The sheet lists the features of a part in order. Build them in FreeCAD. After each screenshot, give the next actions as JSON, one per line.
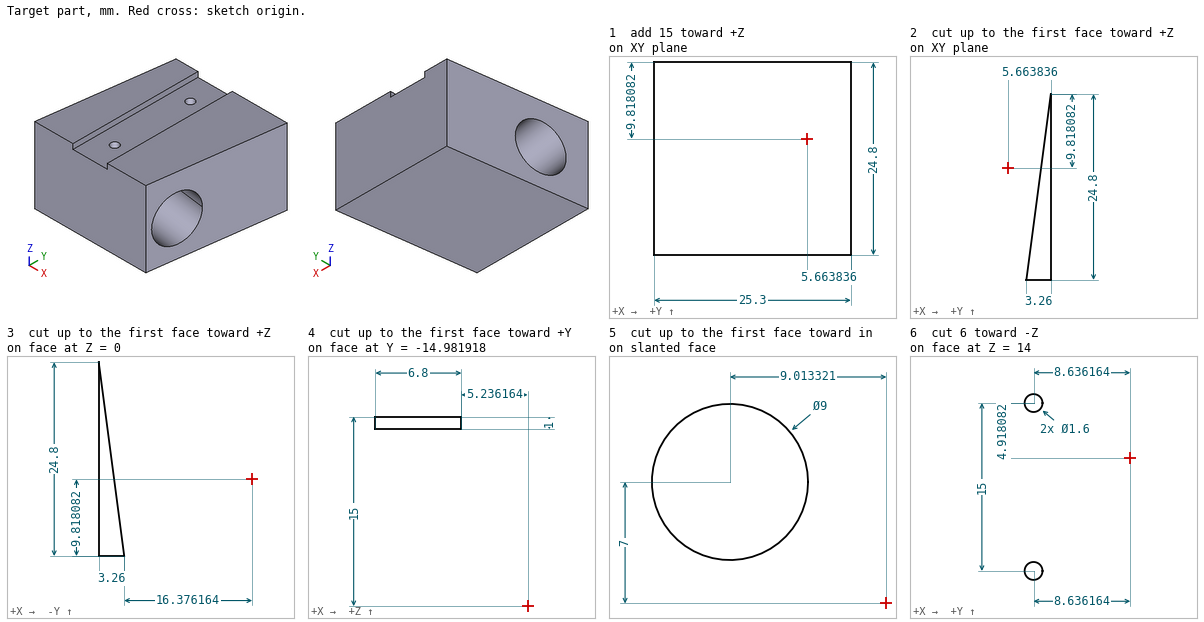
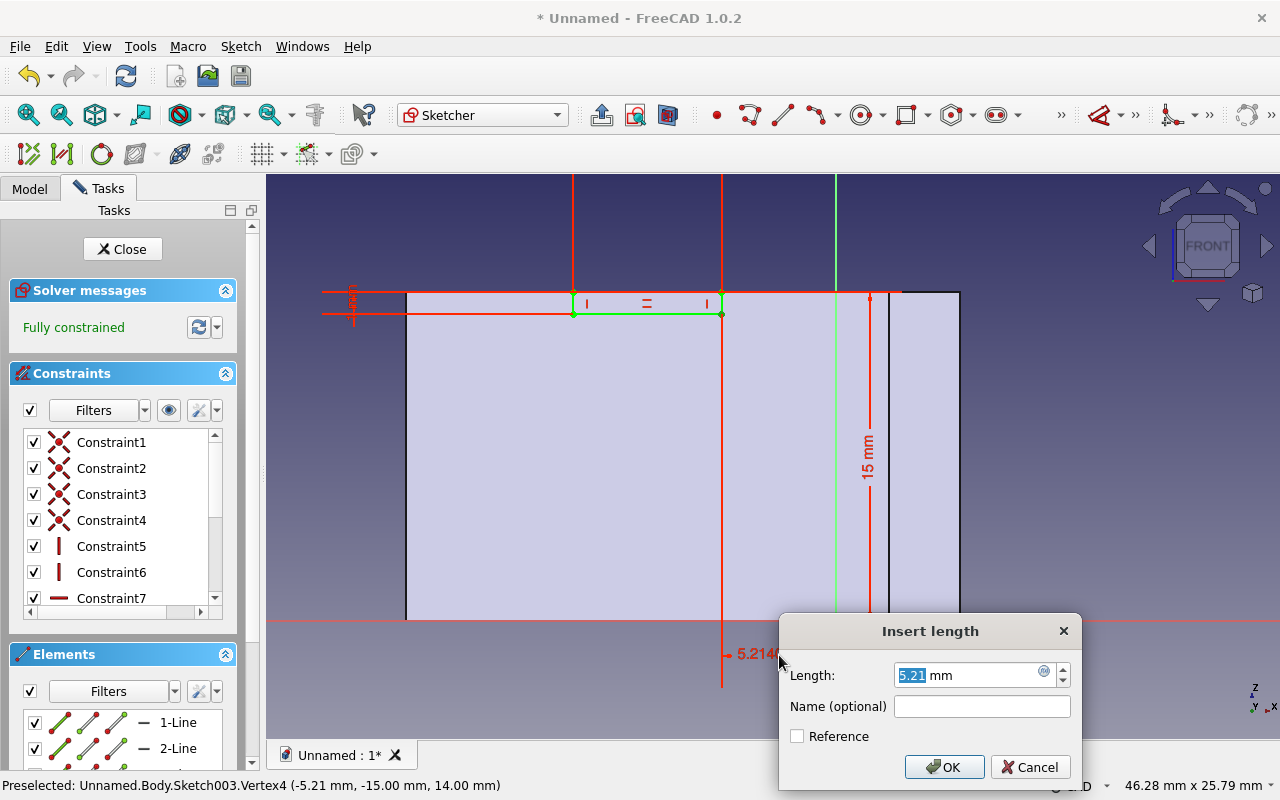
{"action": "type", "text": "5.236164"}
{"action": "key", "text": "Return"}
{"action": "key", "text": "Escape"}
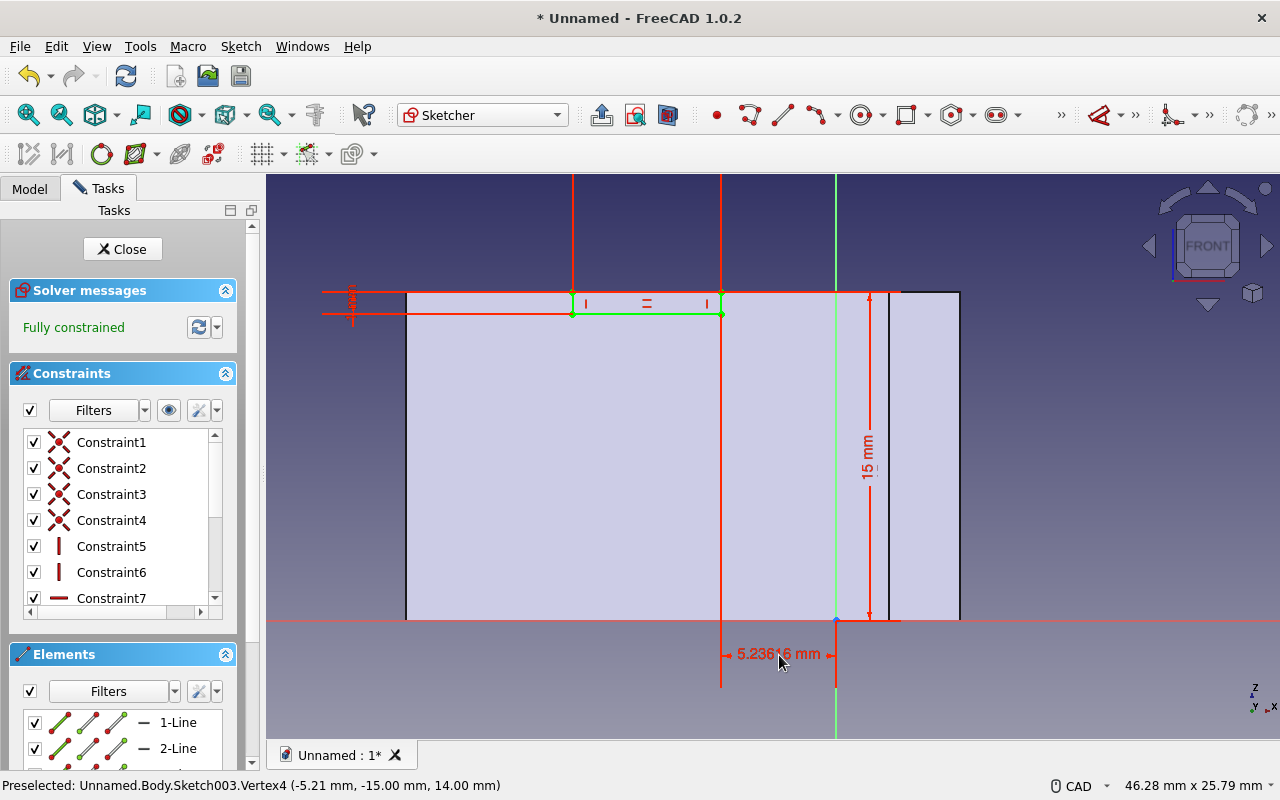
{"action": "left_click", "coordinate": [123, 249]}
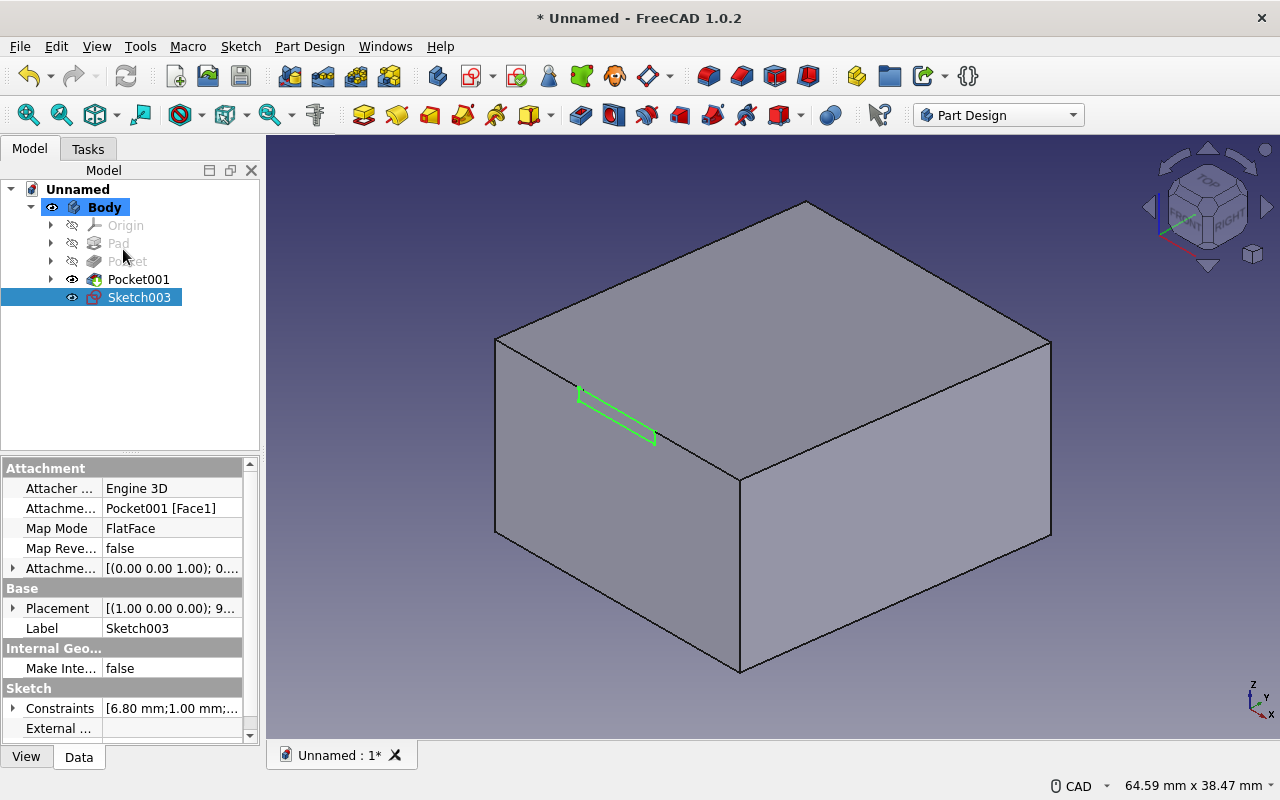
{"action": "left_click", "coordinate": [581, 116]}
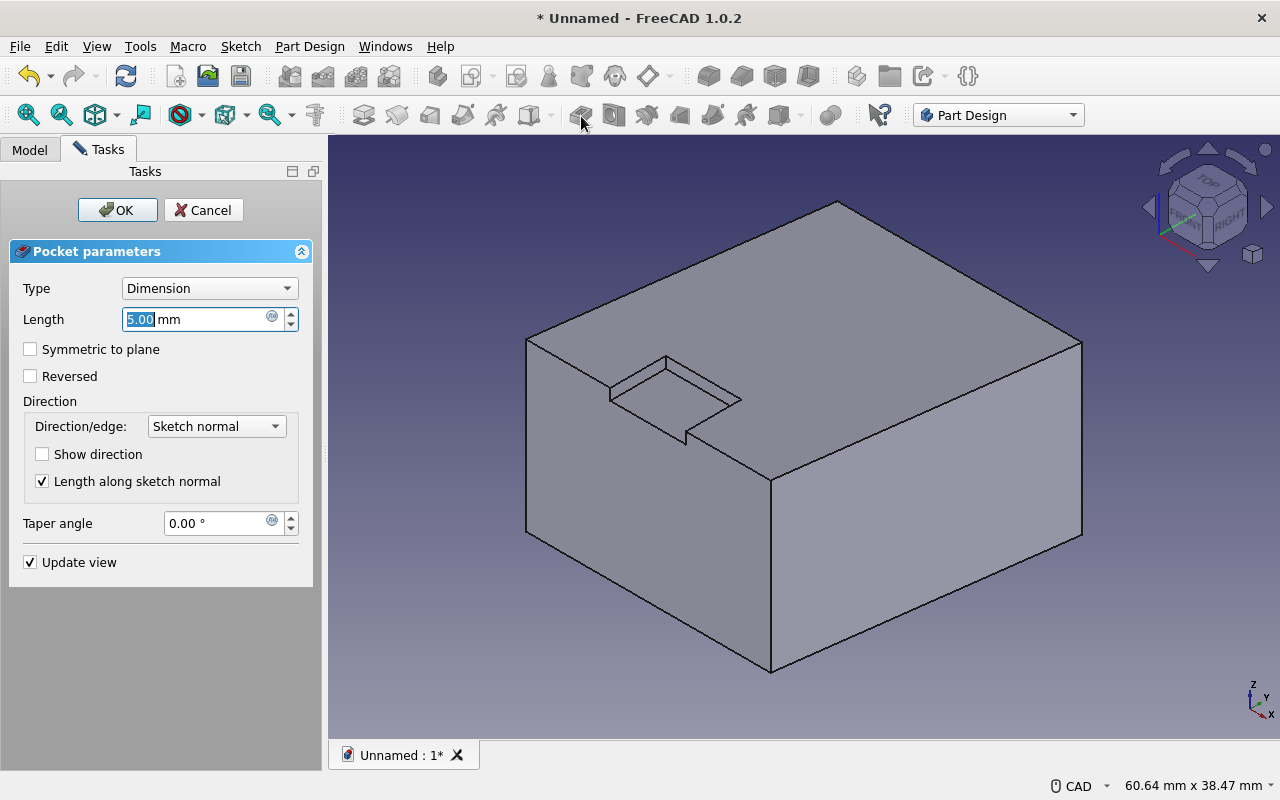
{"action": "left_click", "coordinate": [210, 288]}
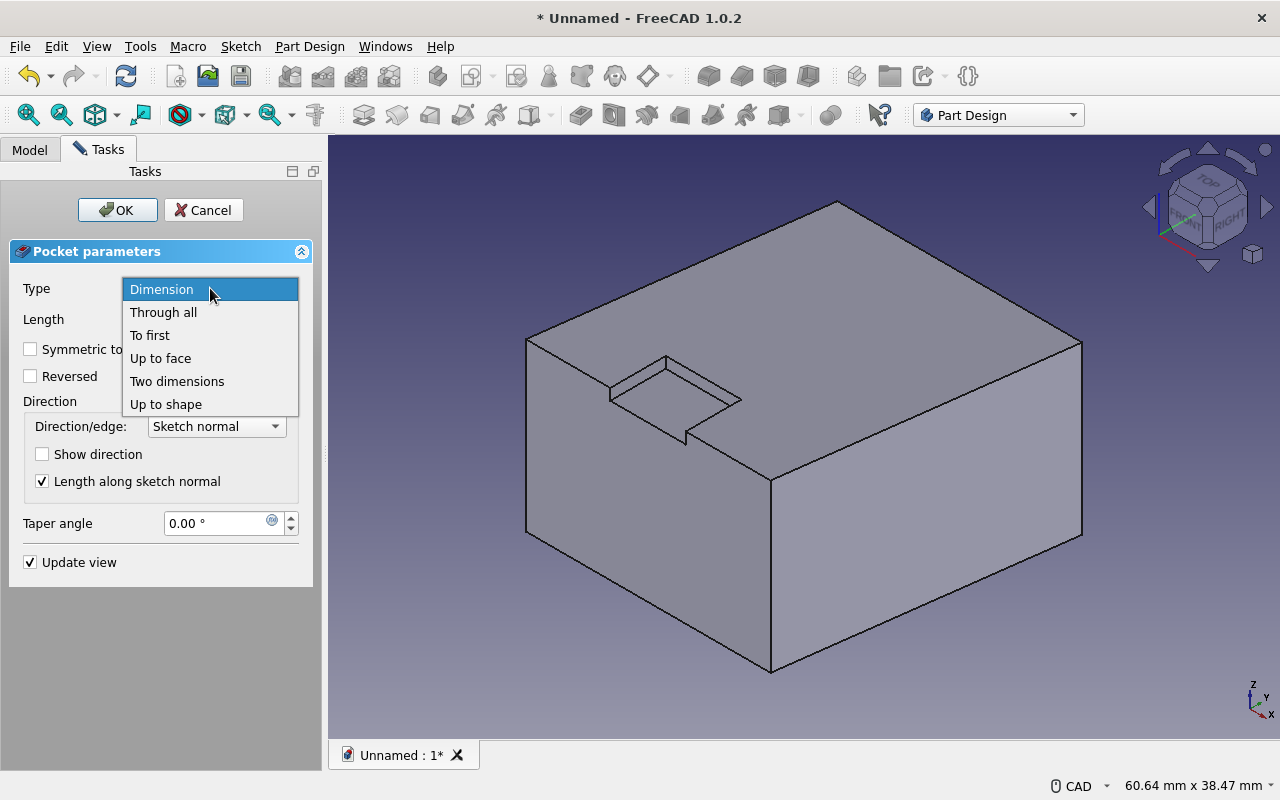
{"action": "left_click", "coordinate": [208, 336]}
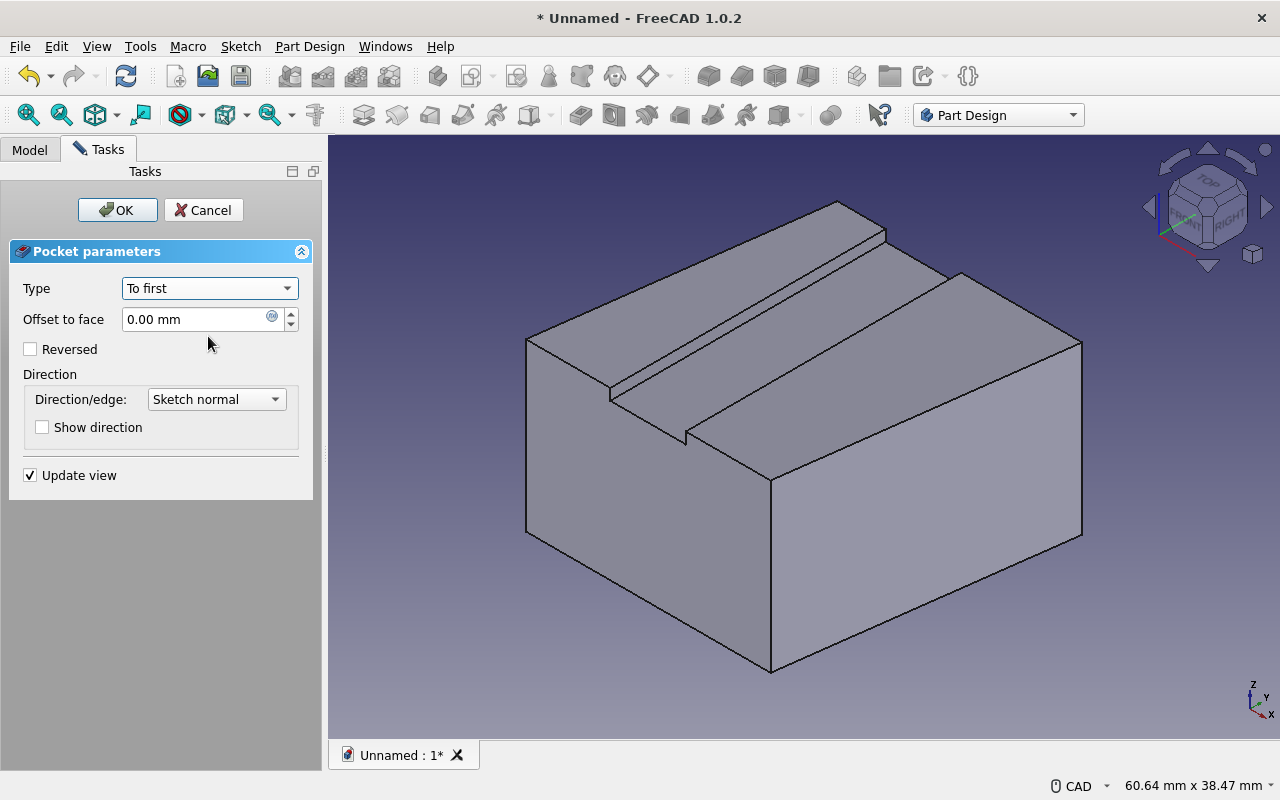
{"action": "left_click", "coordinate": [118, 210]}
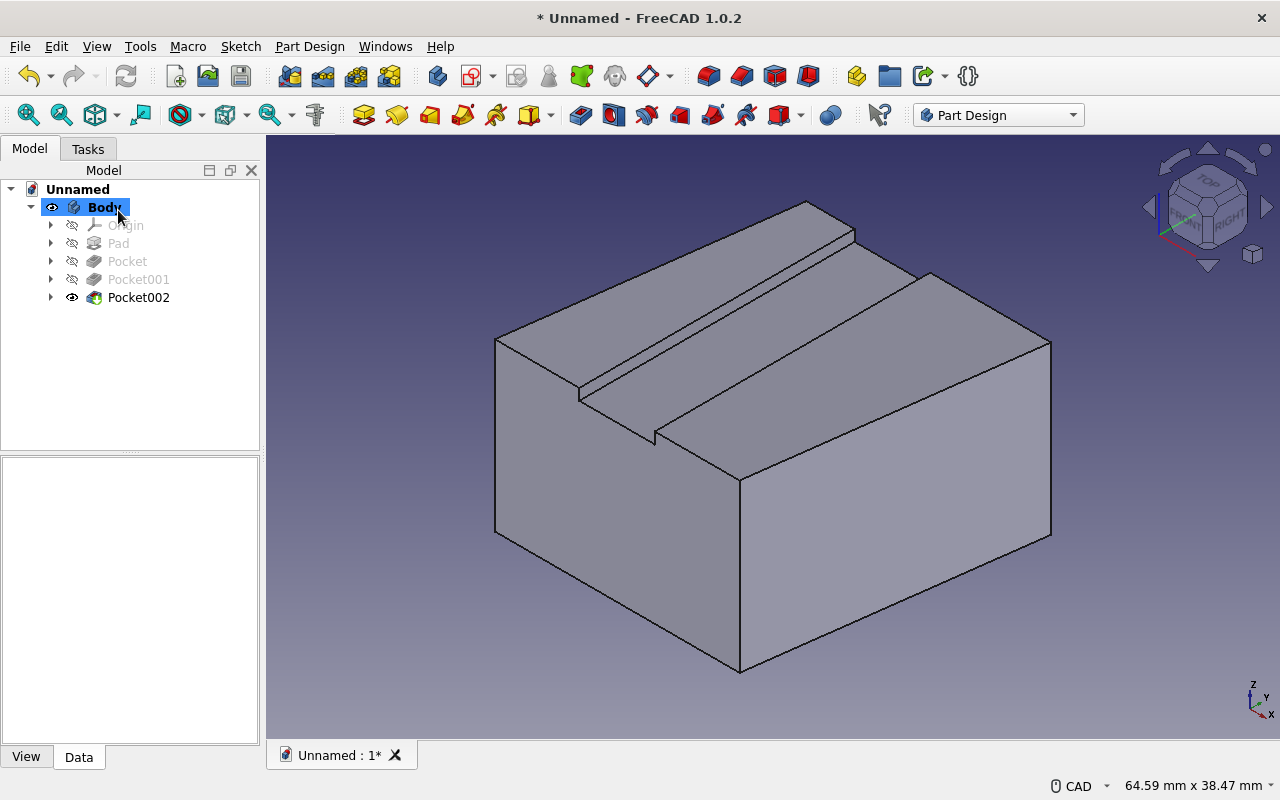
{"action": "left_click", "coordinate": [940, 487]}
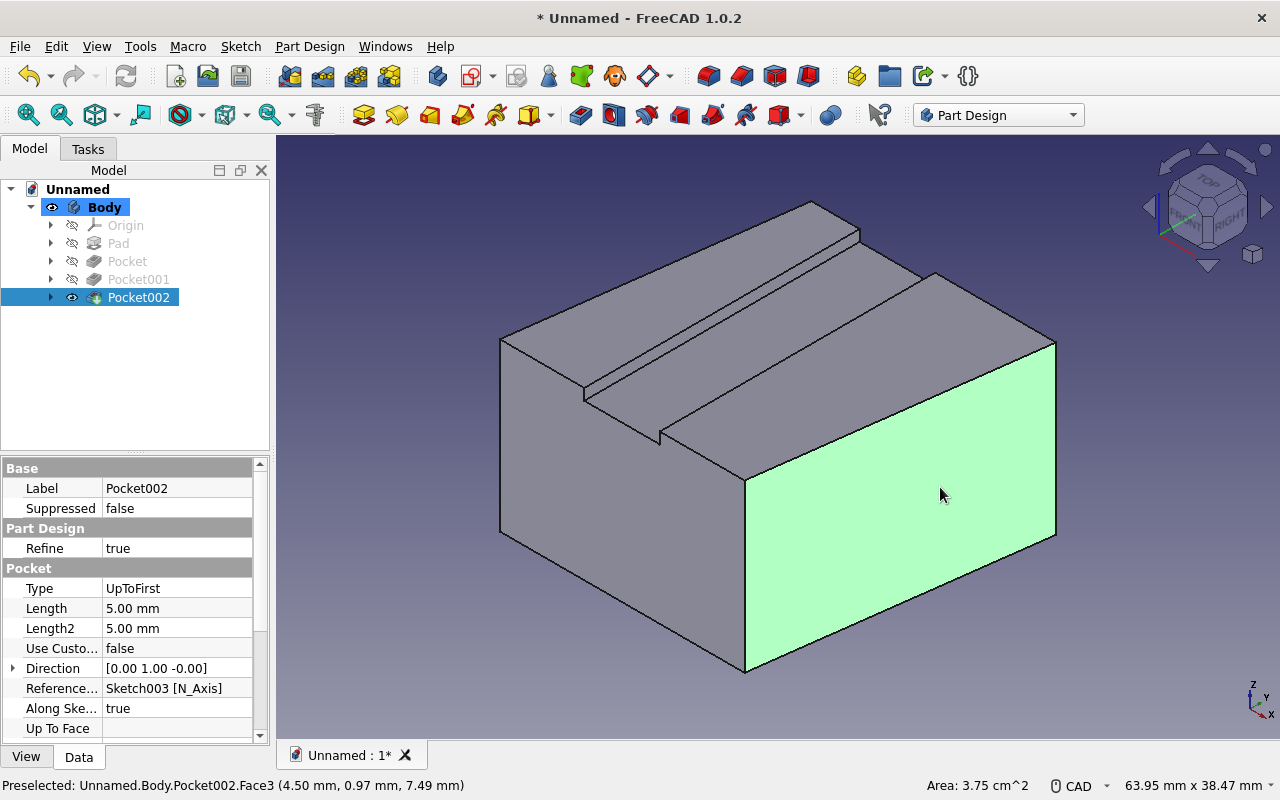
{"action": "left_click", "coordinate": [470, 76]}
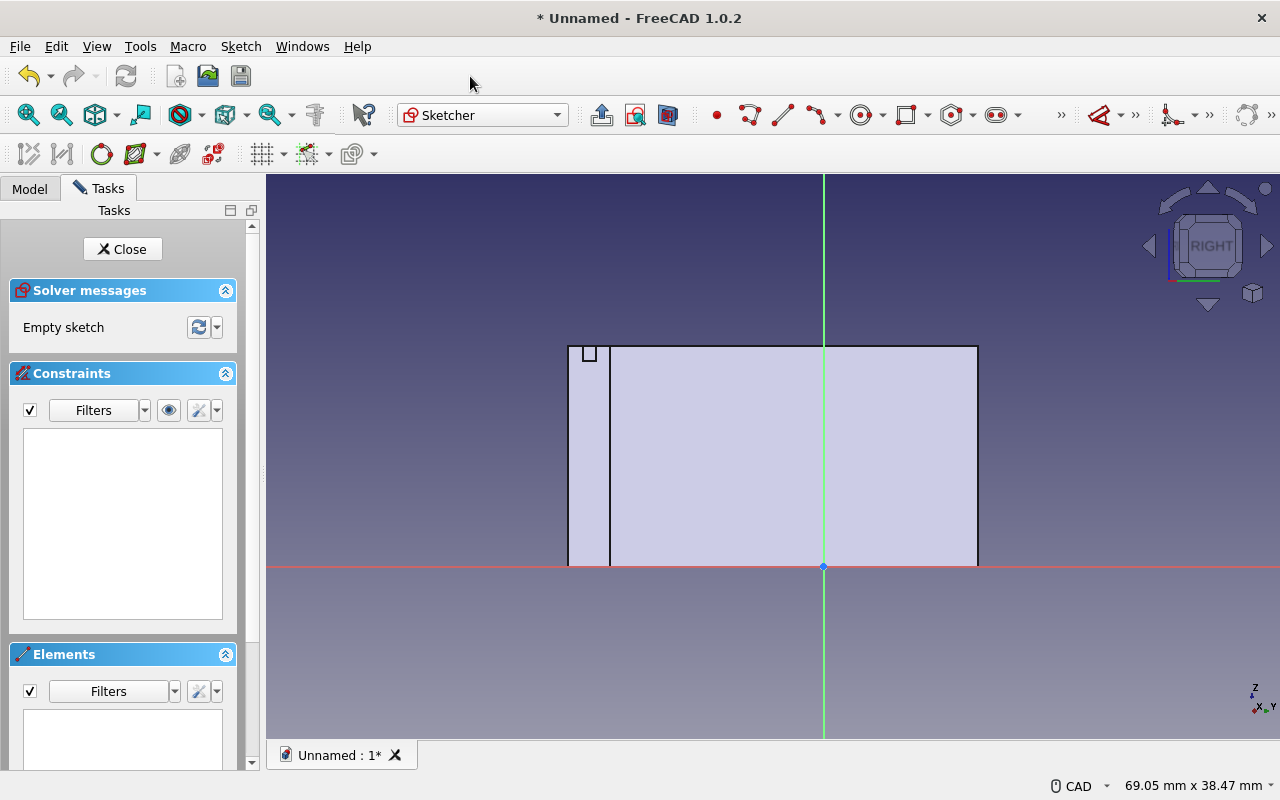
{"action": "left_click", "coordinate": [668, 116]}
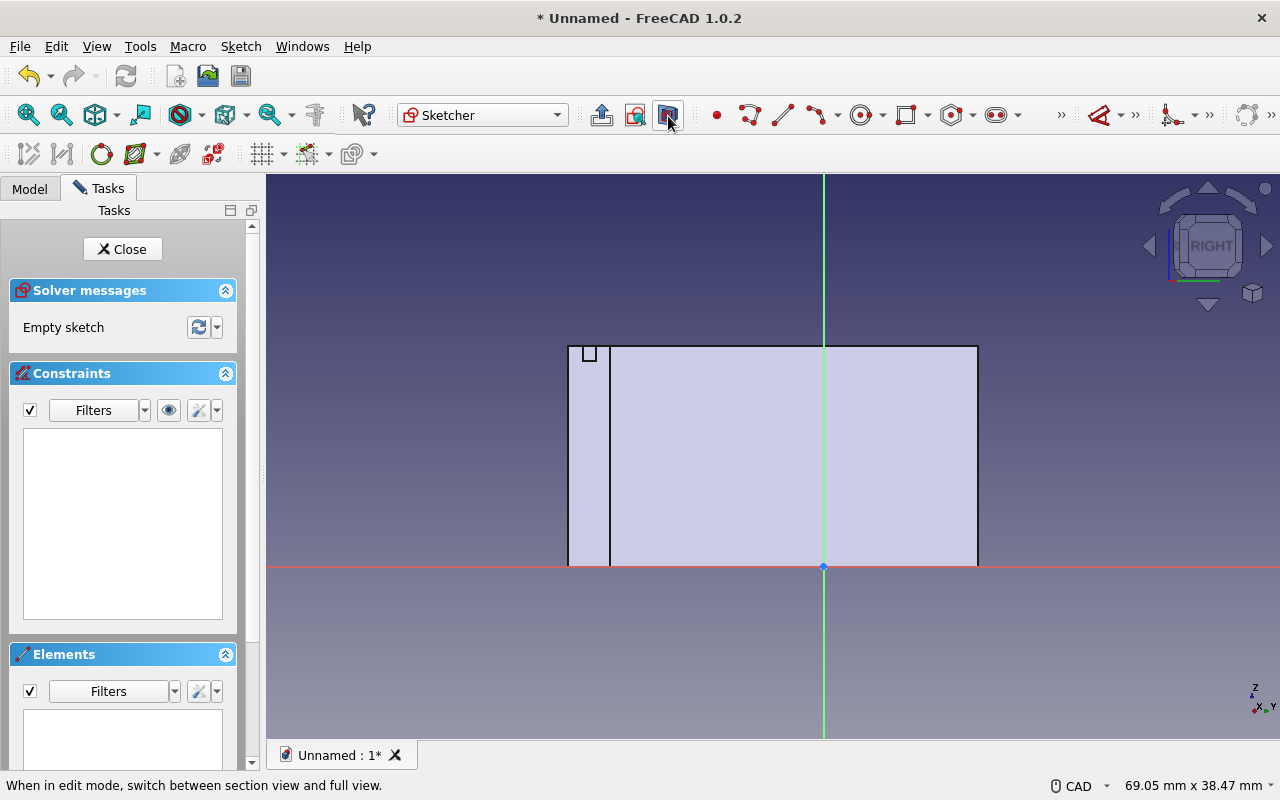
{"action": "scroll", "coordinate": [741, 503], "scroll_direction": "up", "scroll_amount": 4}